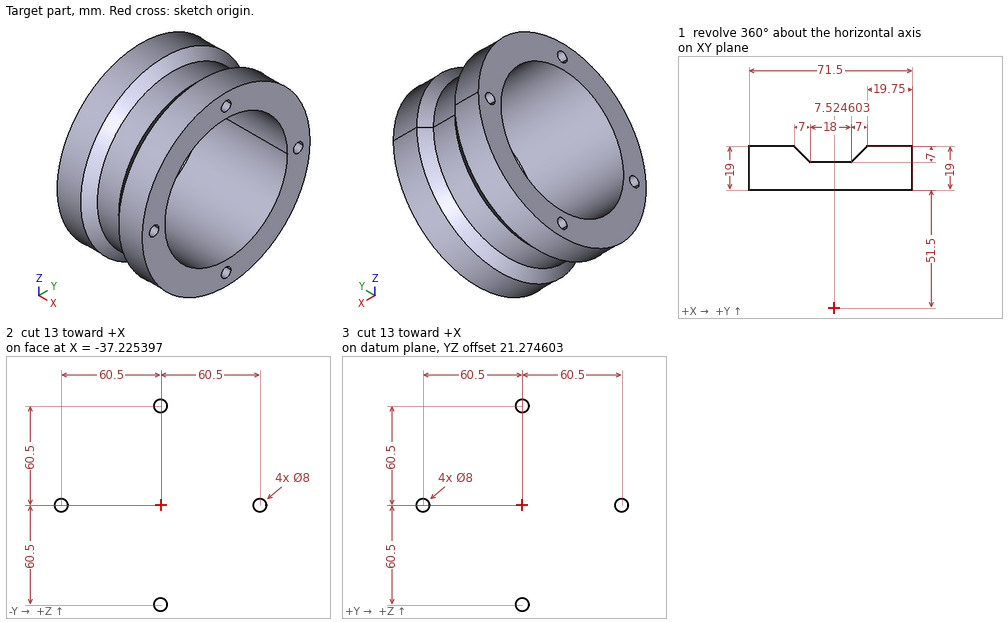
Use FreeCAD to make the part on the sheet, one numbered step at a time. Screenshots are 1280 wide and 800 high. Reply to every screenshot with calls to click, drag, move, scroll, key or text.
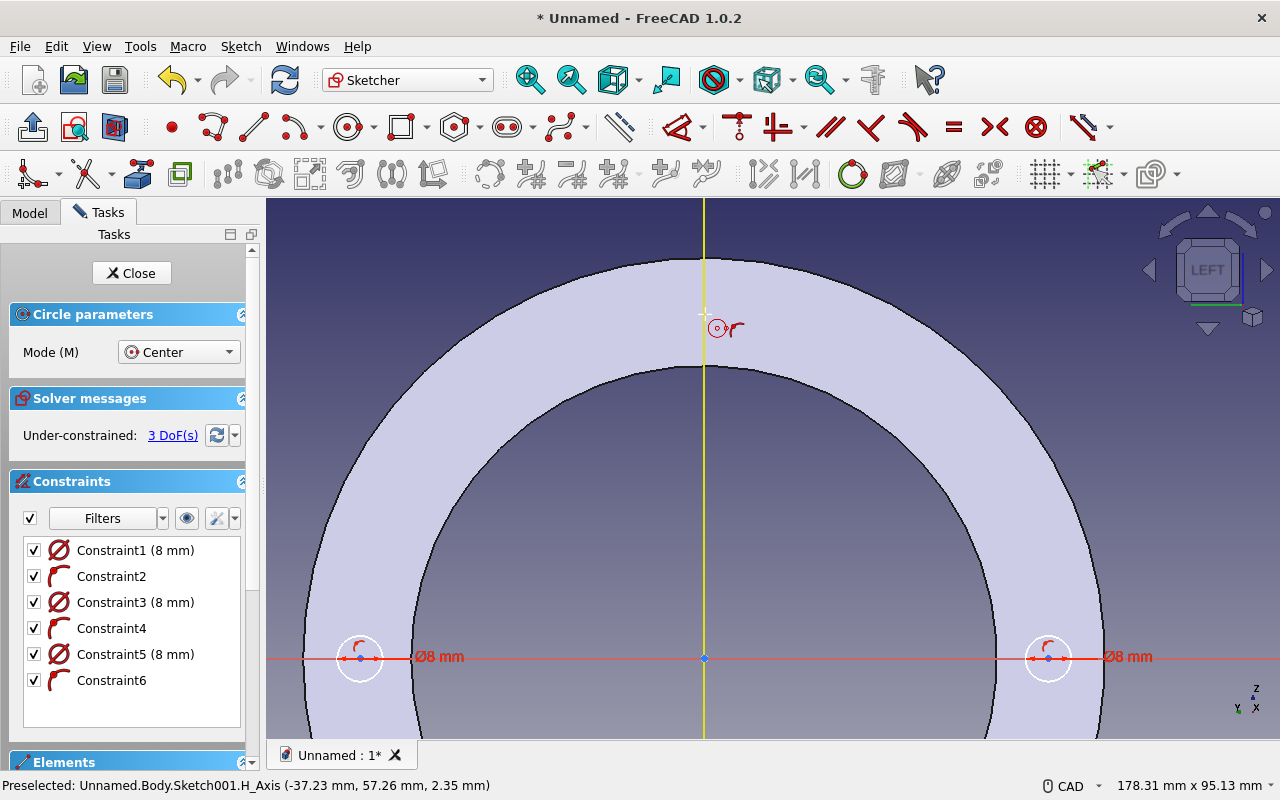
click(704, 315)
move(720, 299)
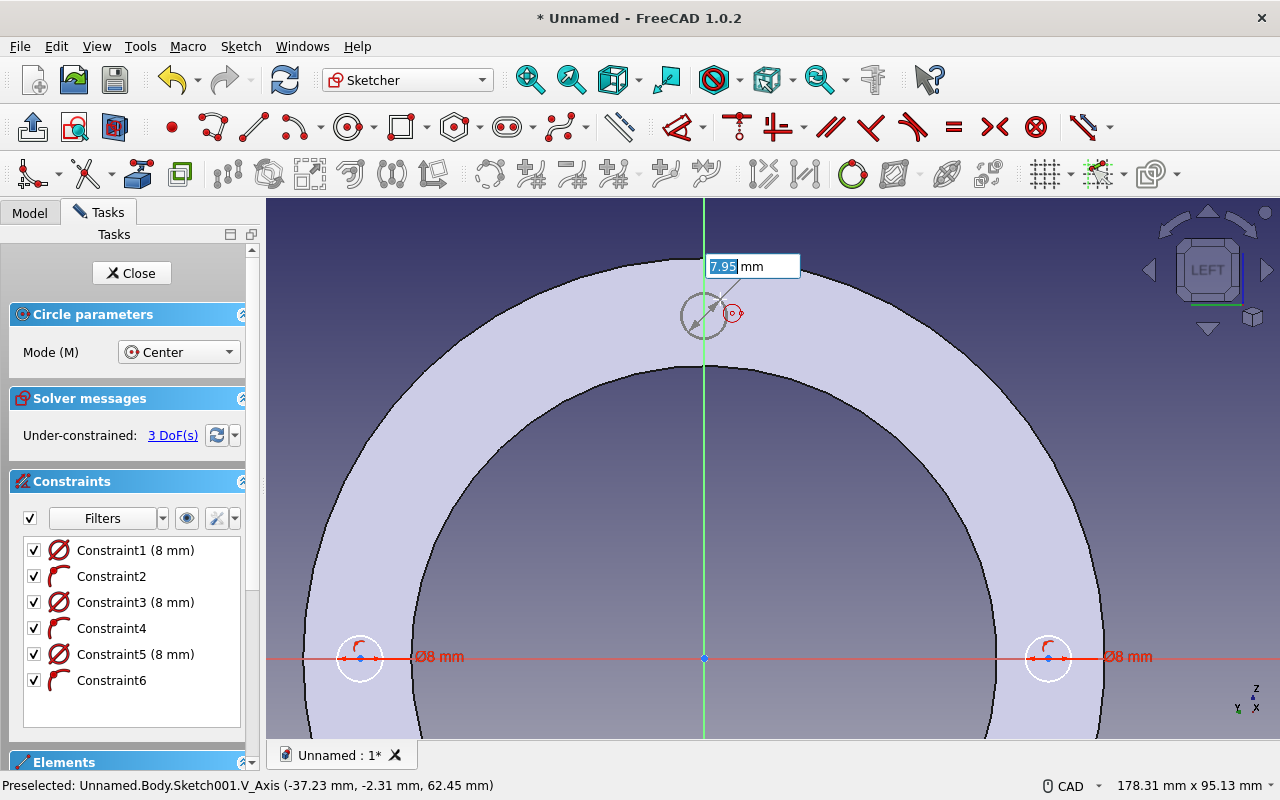
text(8)
key(Return)
key(Escape)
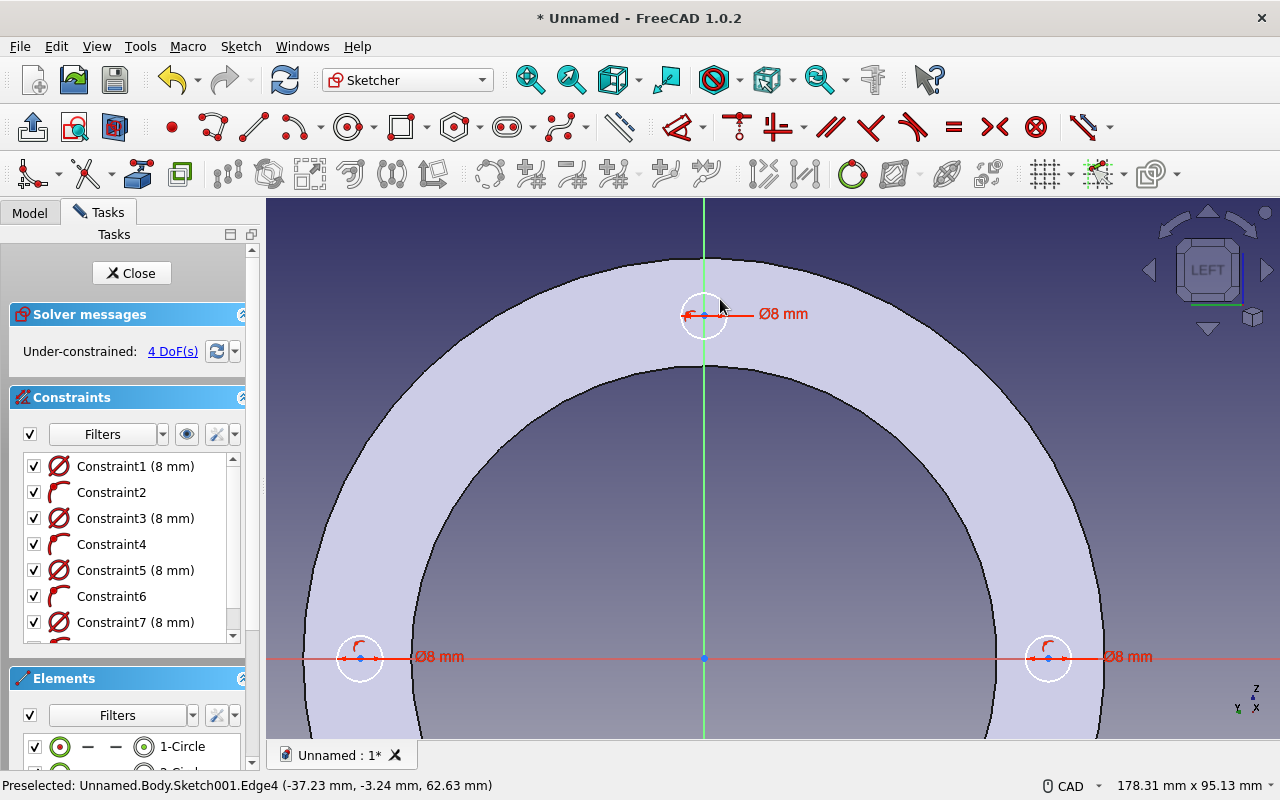
click(676, 128)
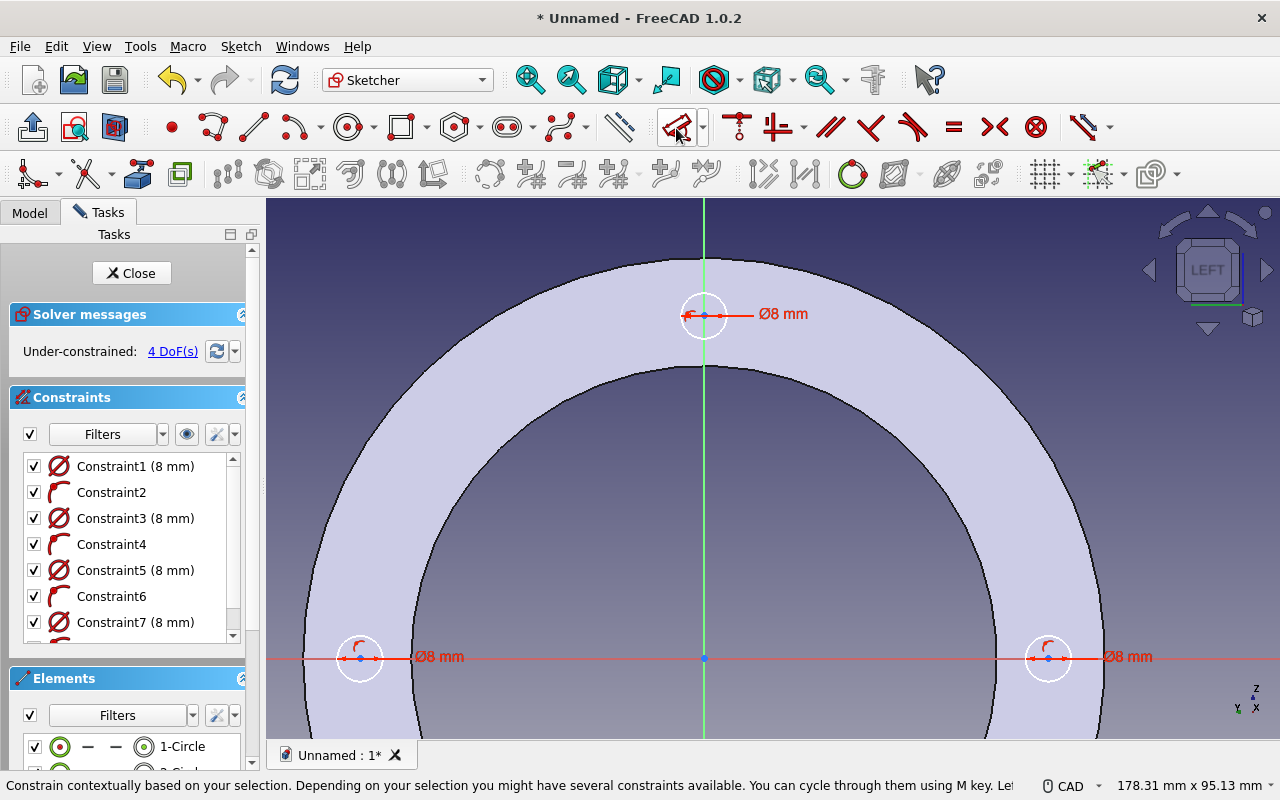
click(1048, 659)
click(876, 693)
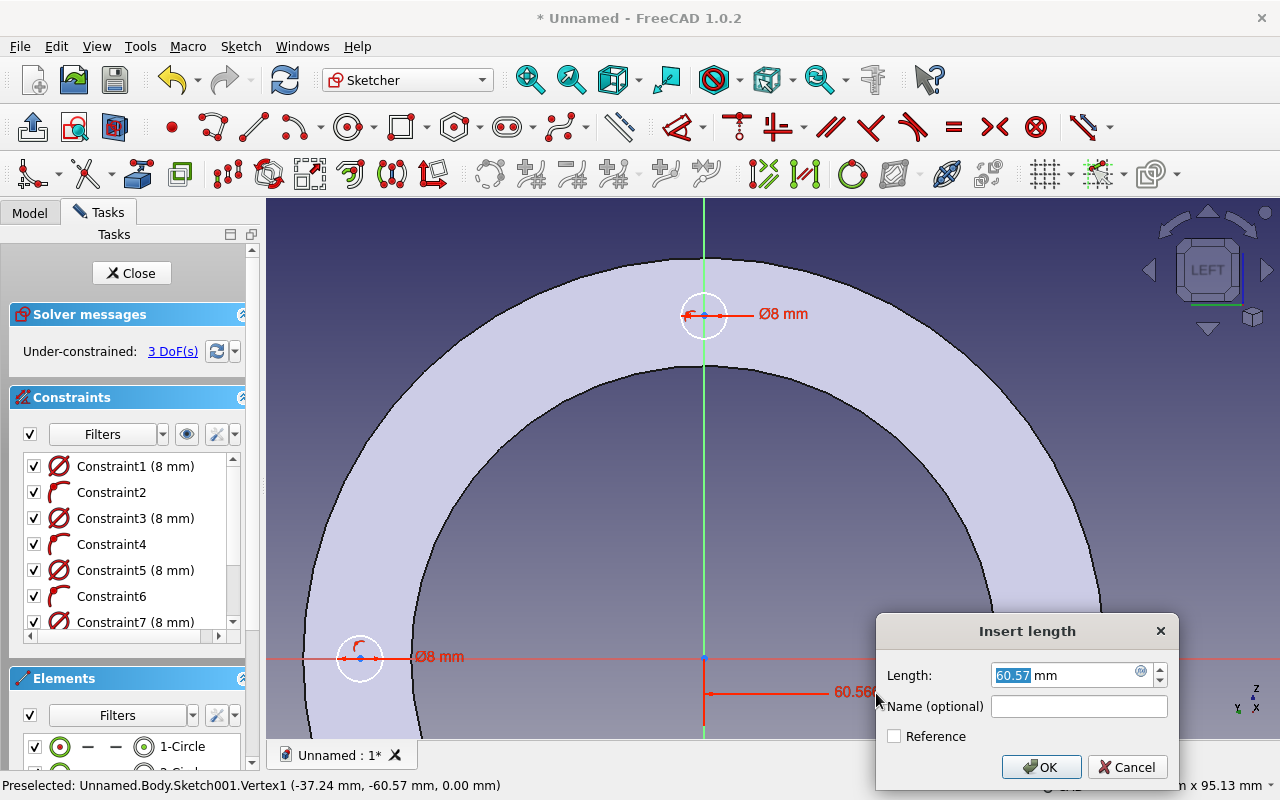
text(60.5)
key(Return)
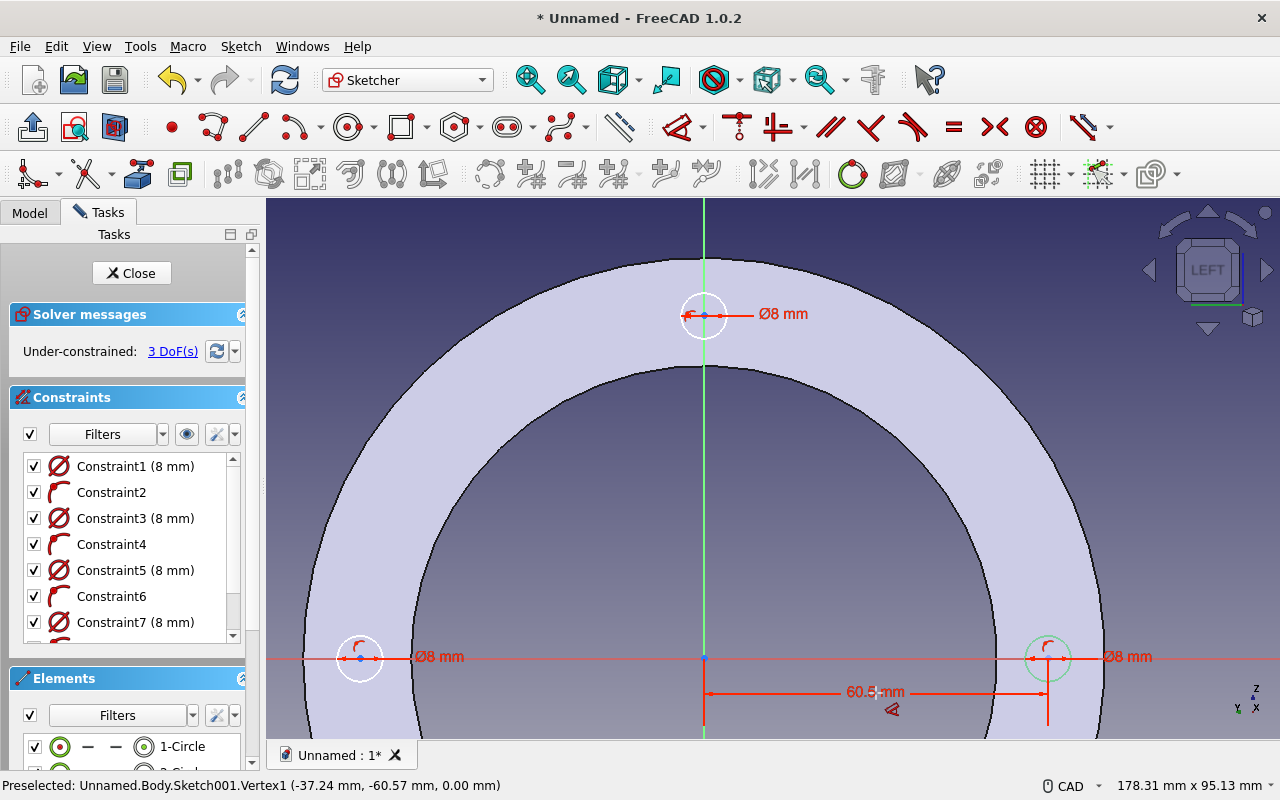
scroll(705, 313, down, 4)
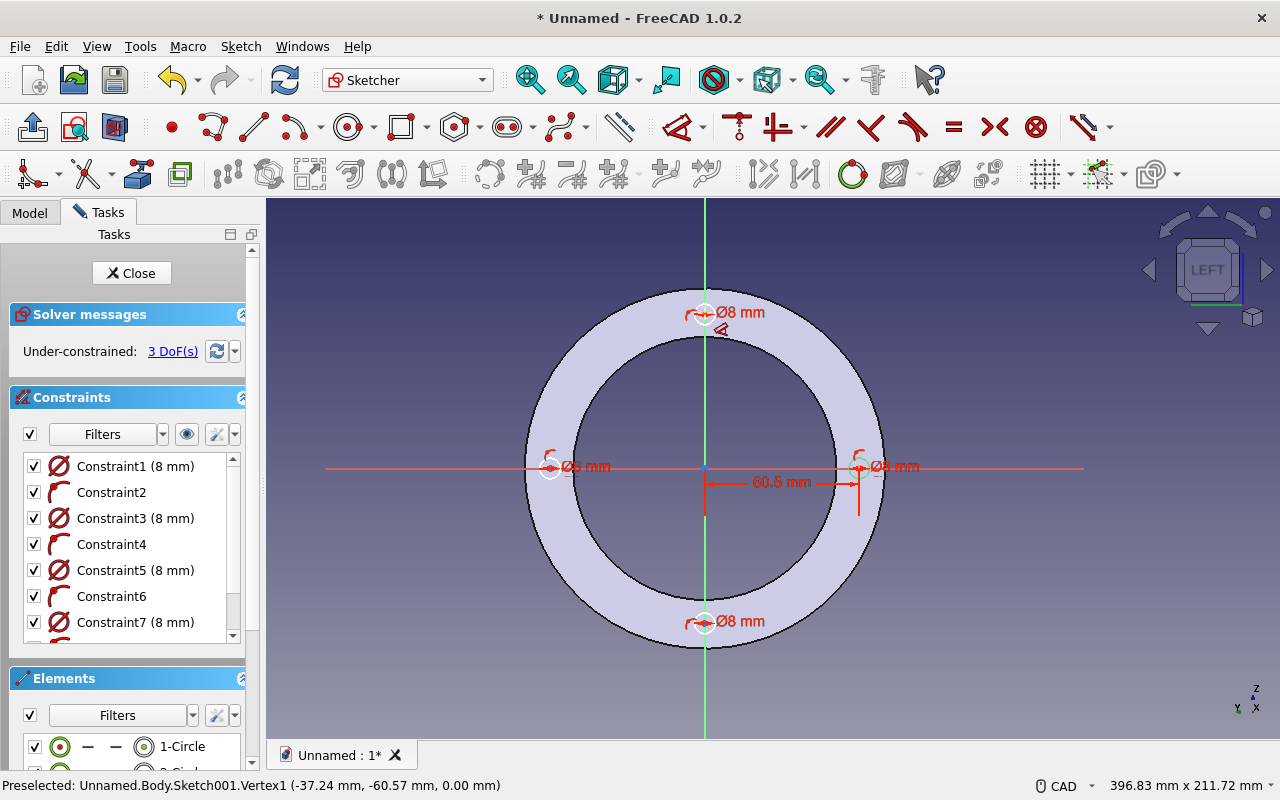
click(705, 623)
click(739, 546)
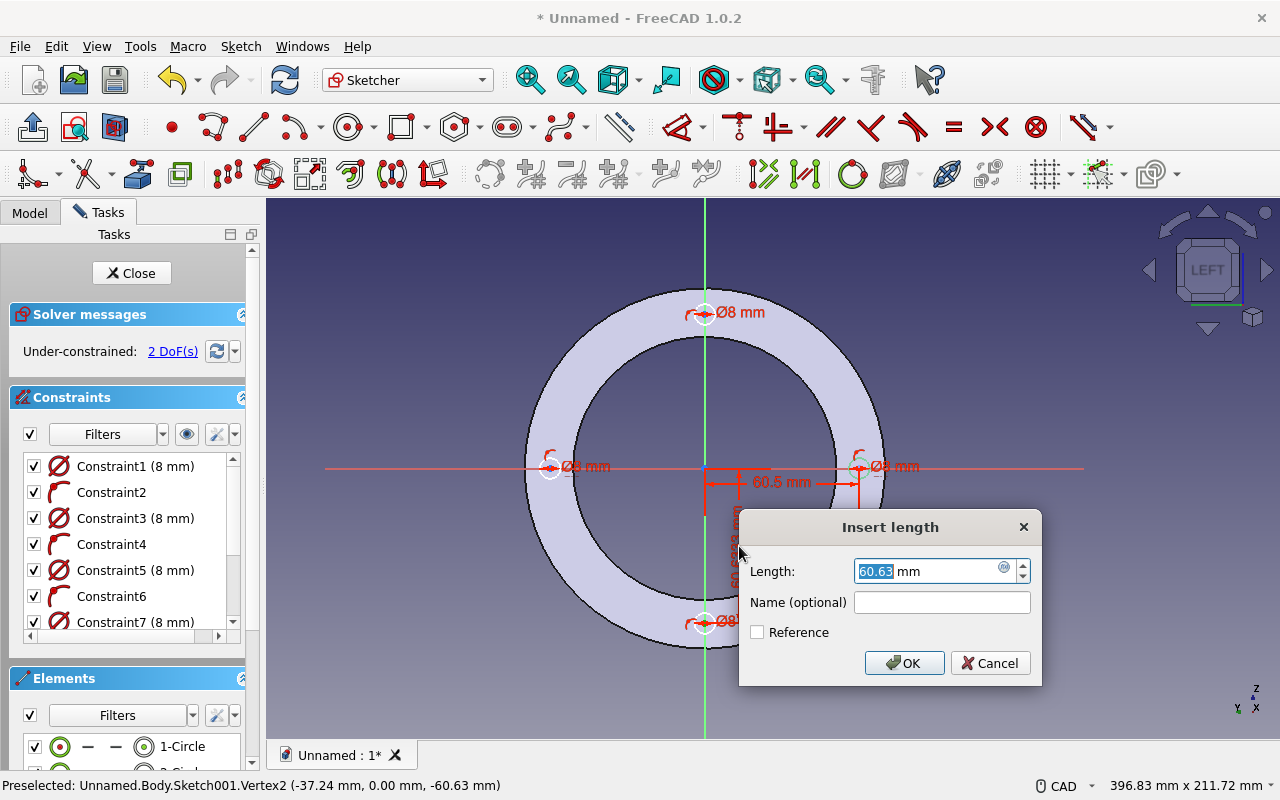
text(60.5)
key(Return)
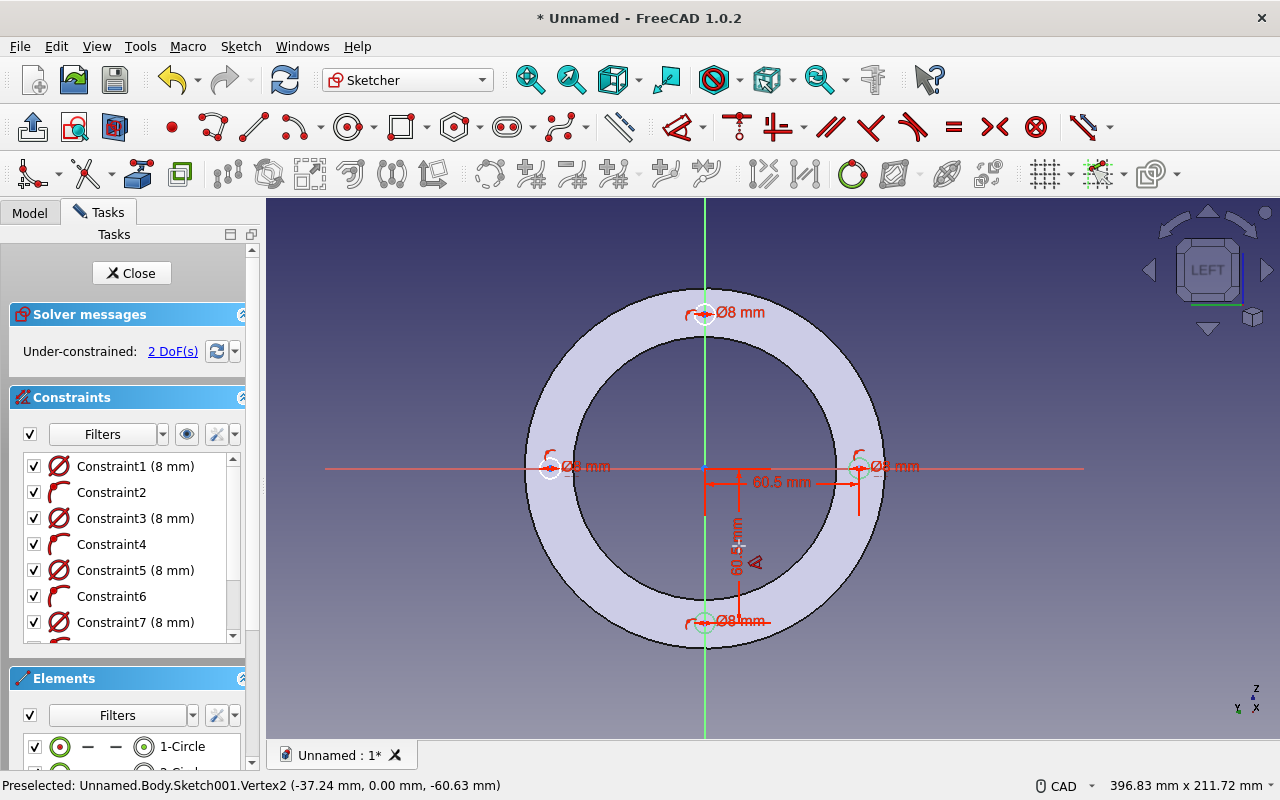
click(550, 468)
click(628, 502)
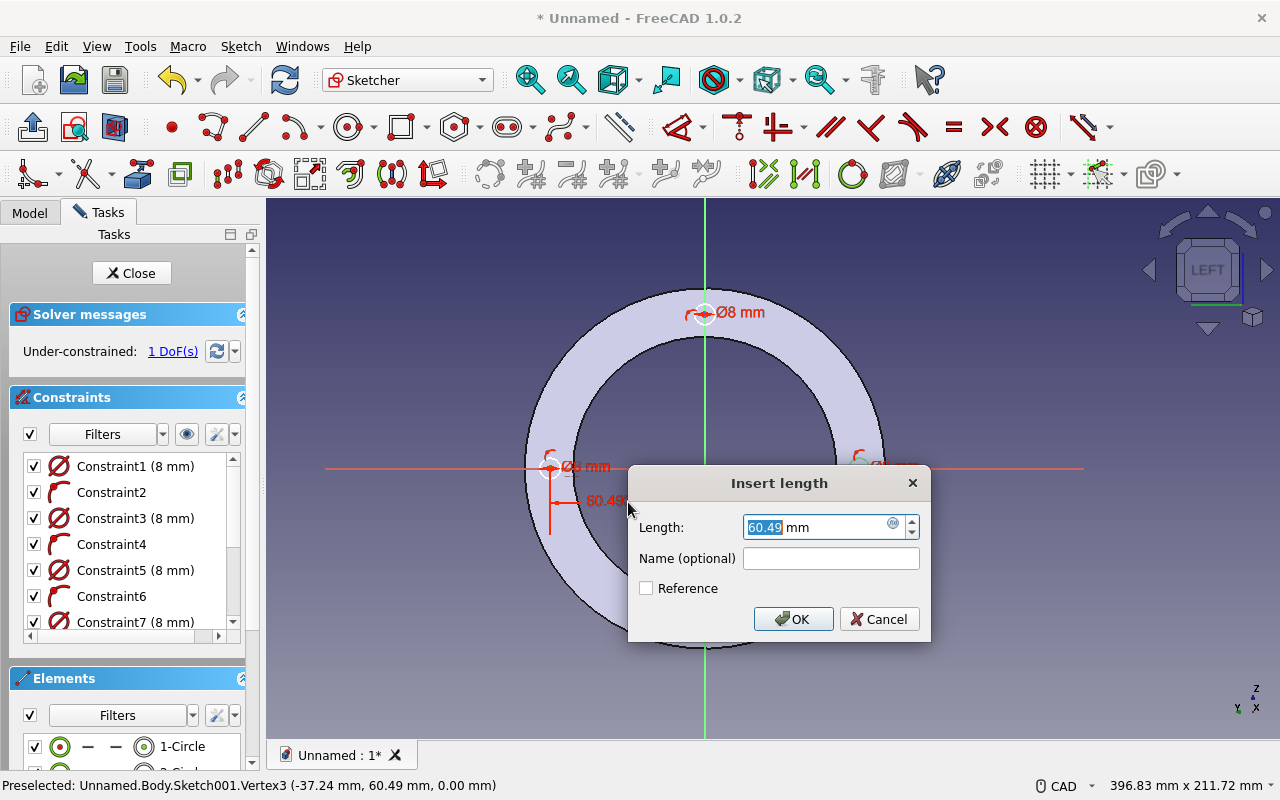
text(60.5)
key(Return)